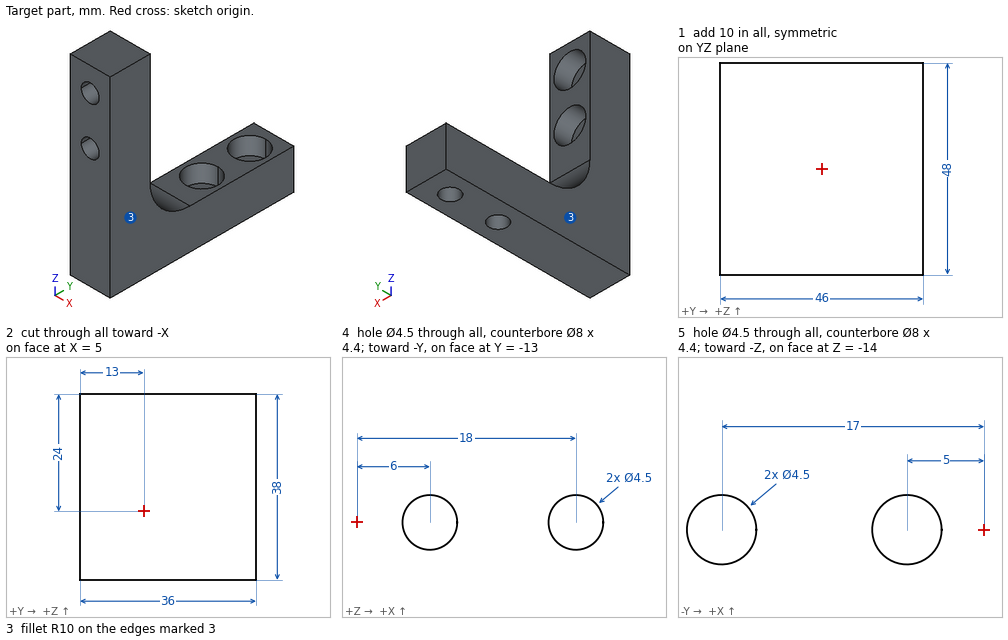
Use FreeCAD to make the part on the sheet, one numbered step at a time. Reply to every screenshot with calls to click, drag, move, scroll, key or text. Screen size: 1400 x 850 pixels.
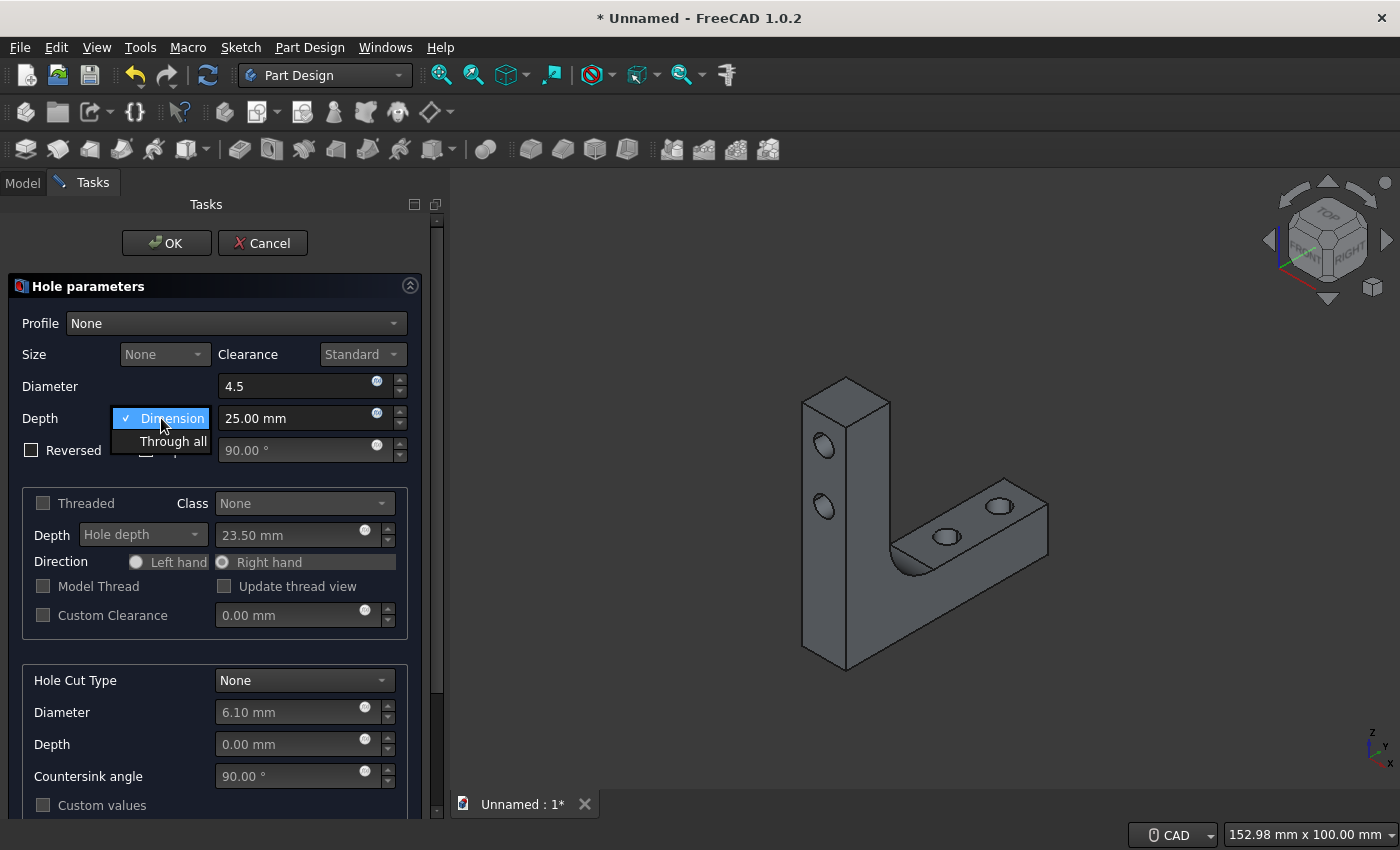
click(160, 442)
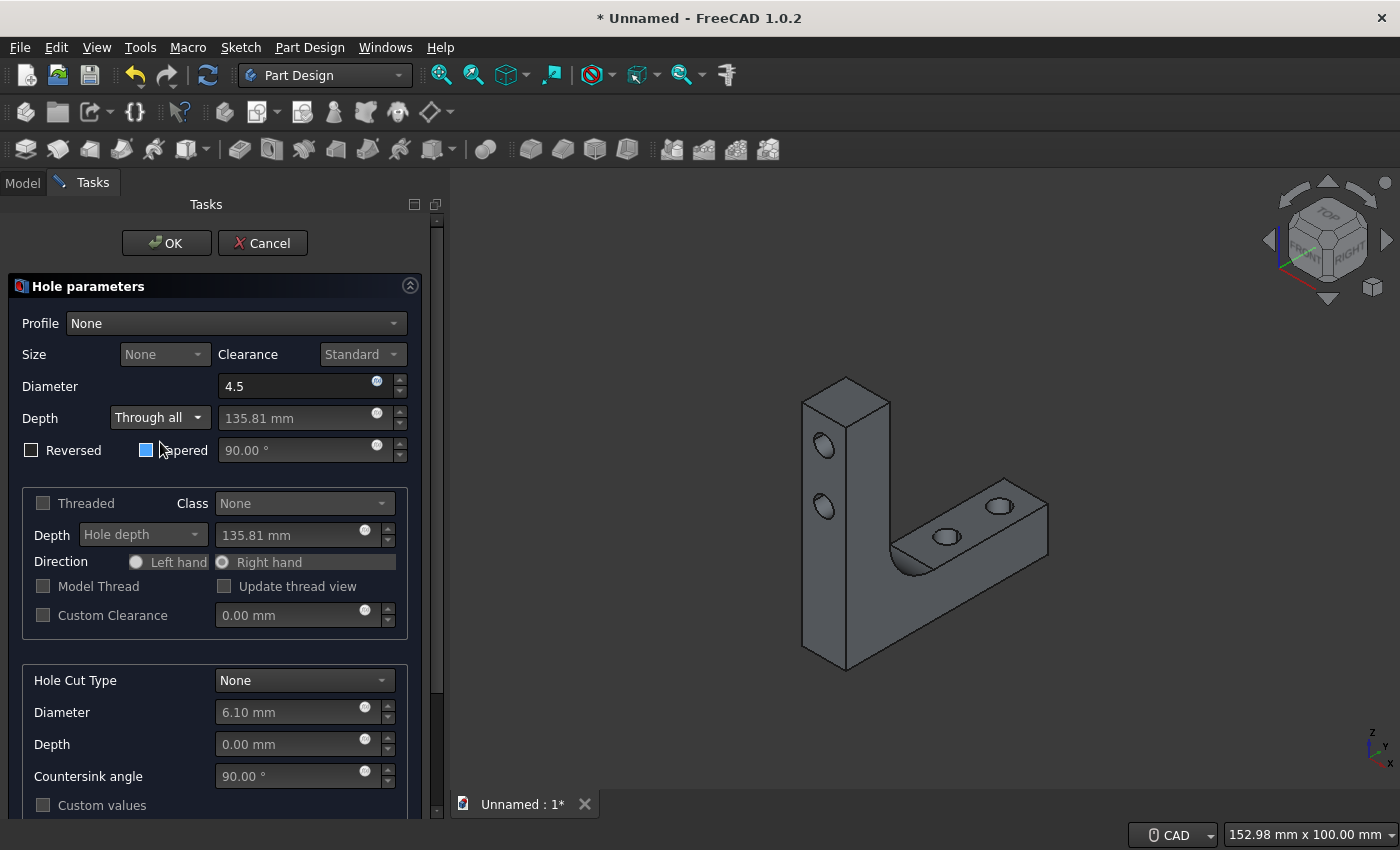
click(306, 680)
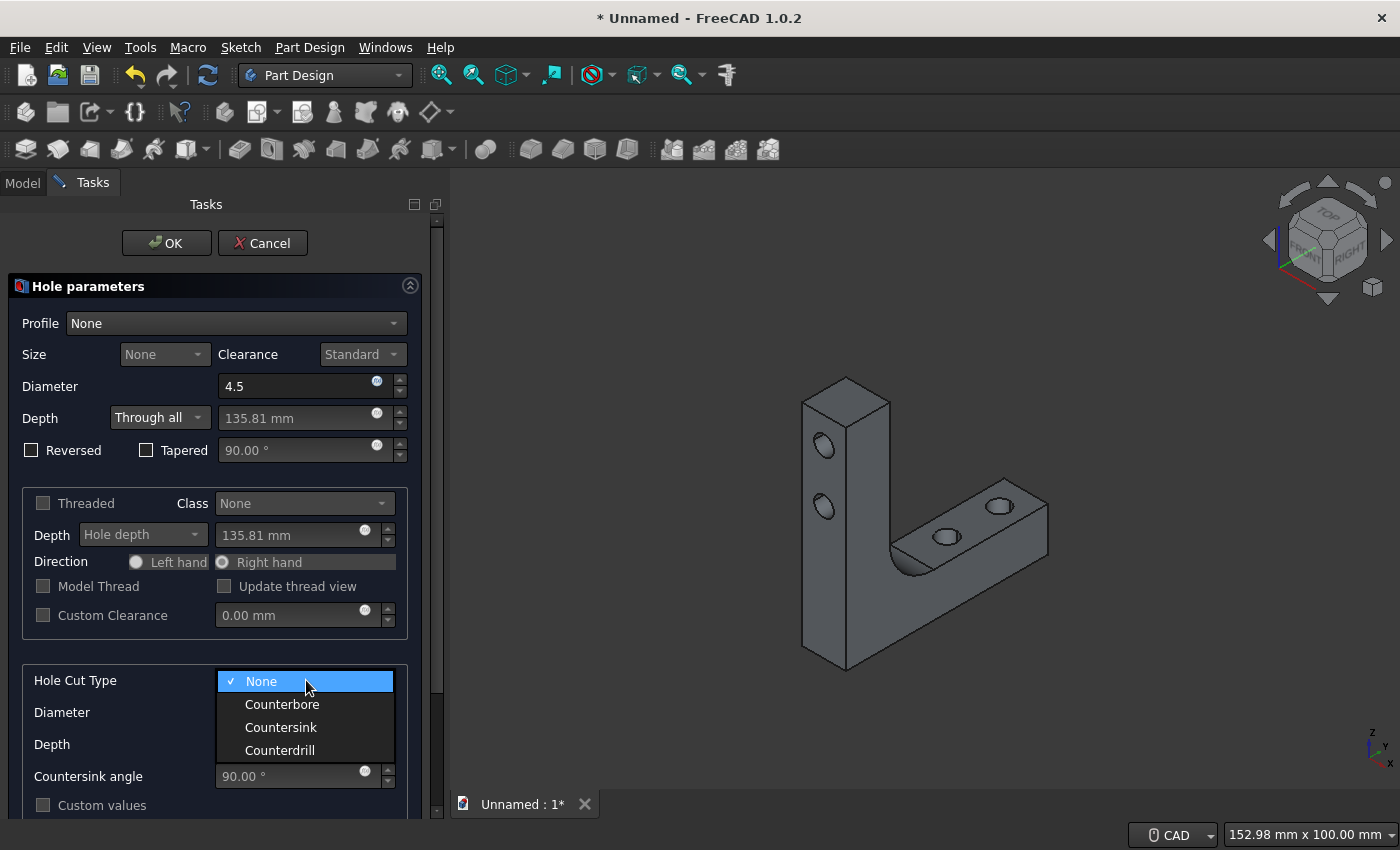
click(304, 704)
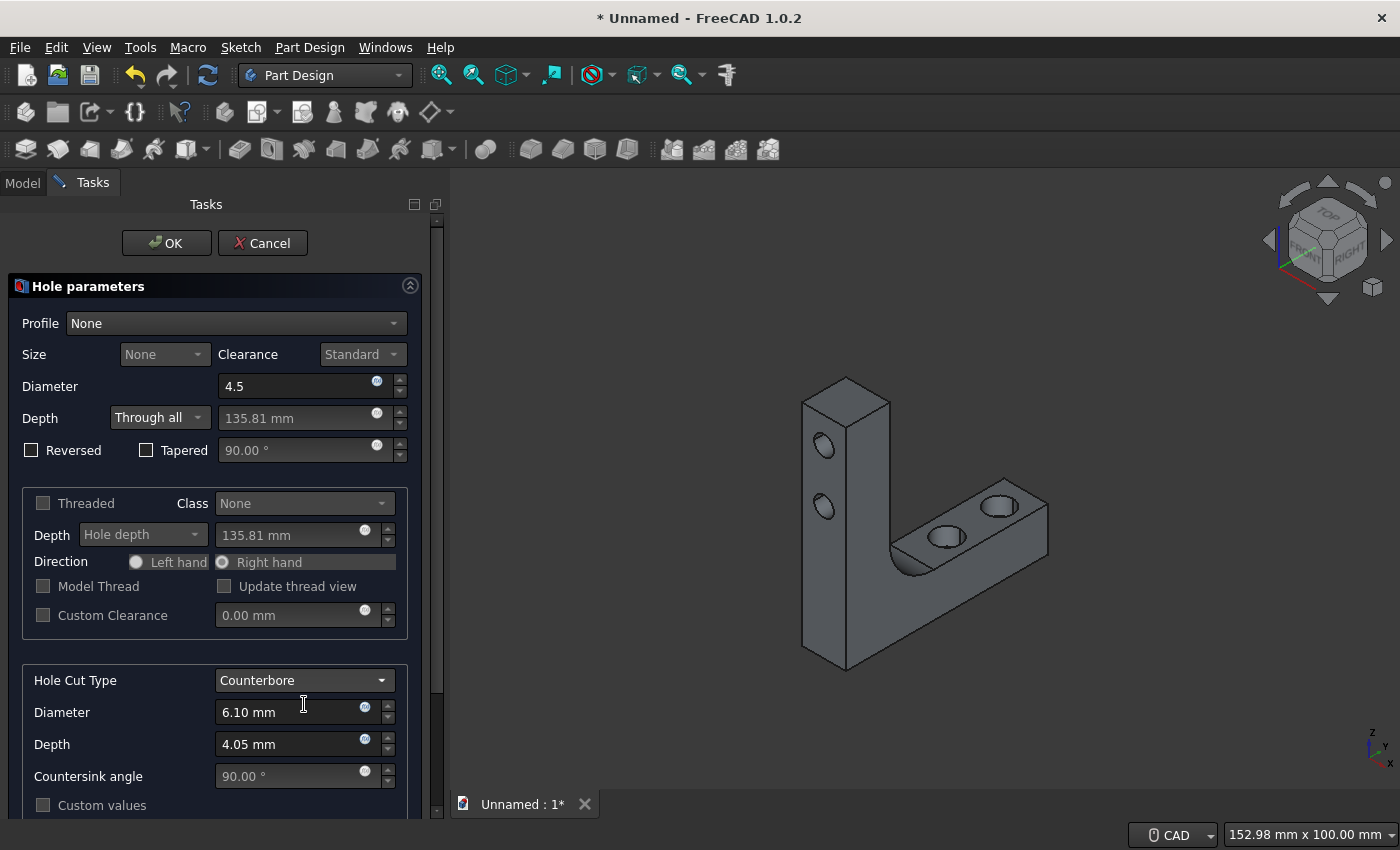
triple_click(298, 712)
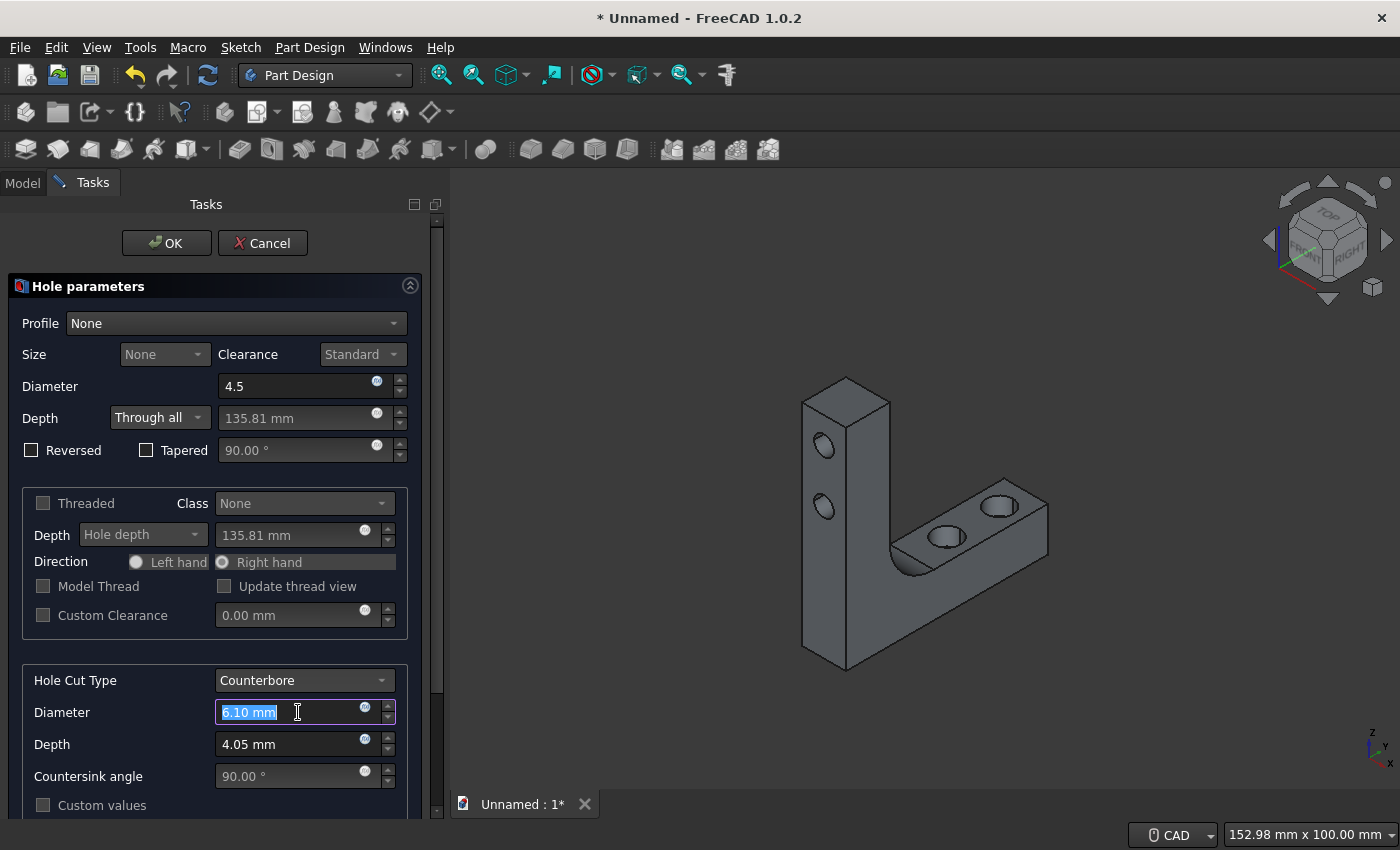
text(8)
key(Tab)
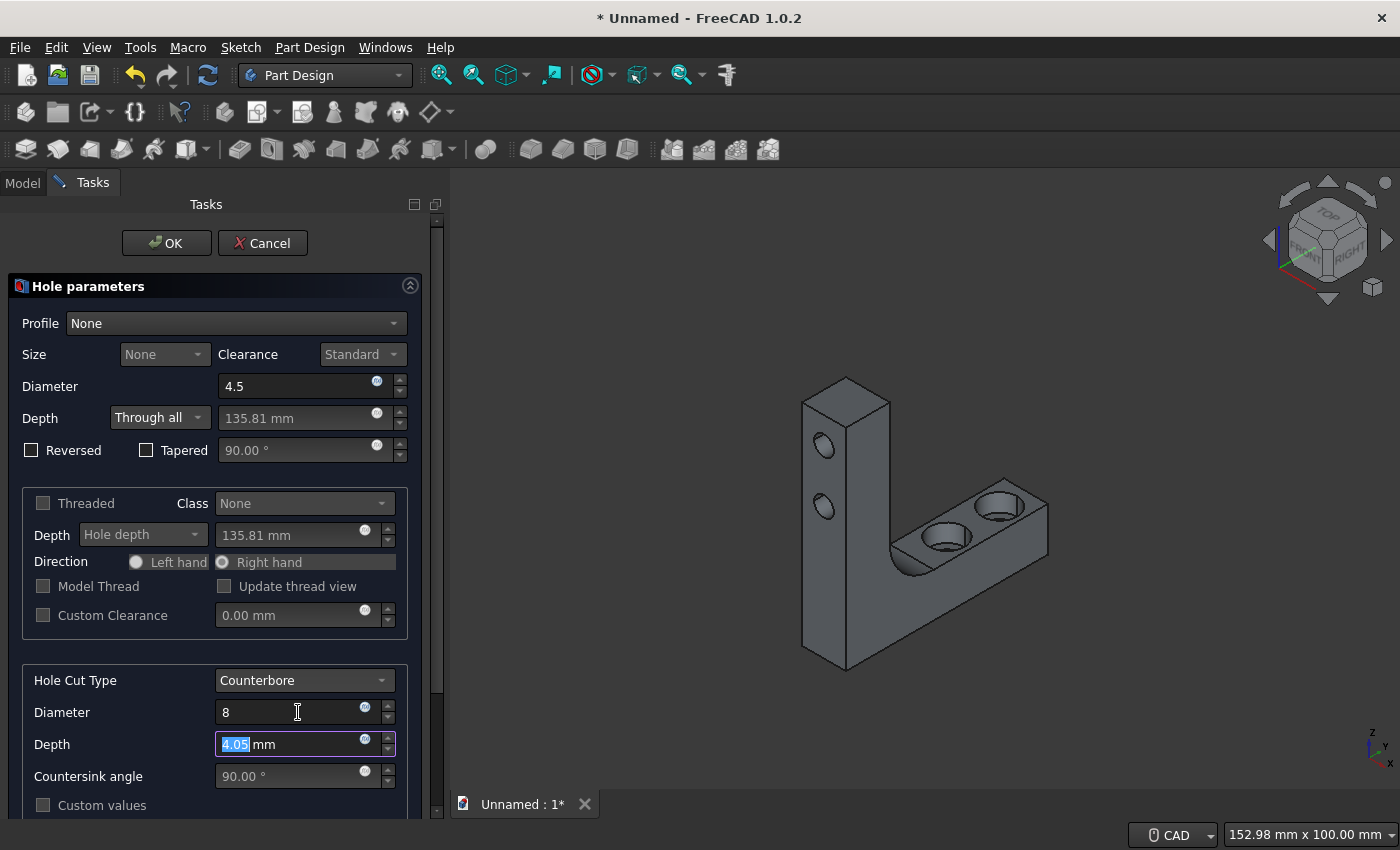
text(4.4)
key(Tab)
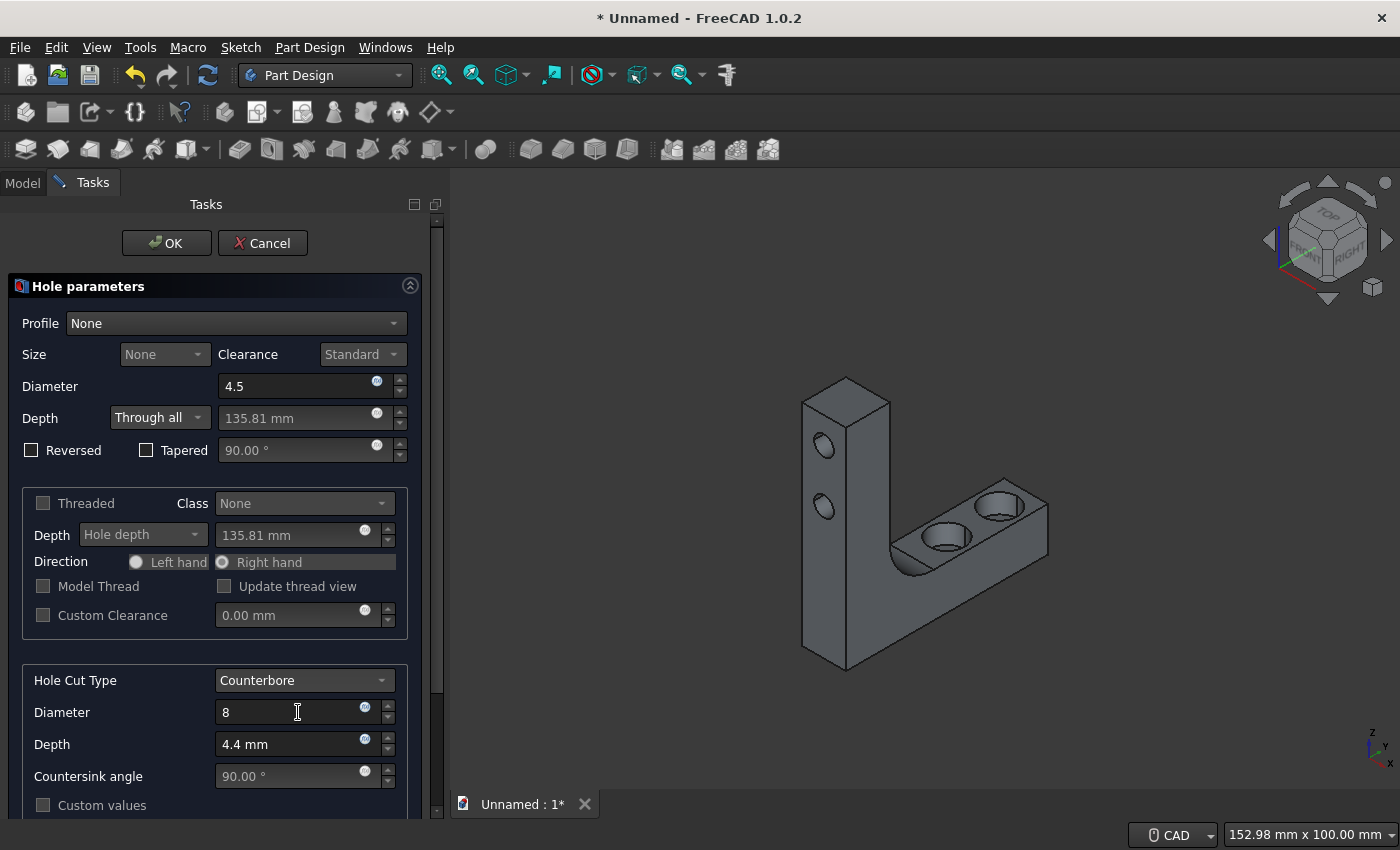
click(167, 243)